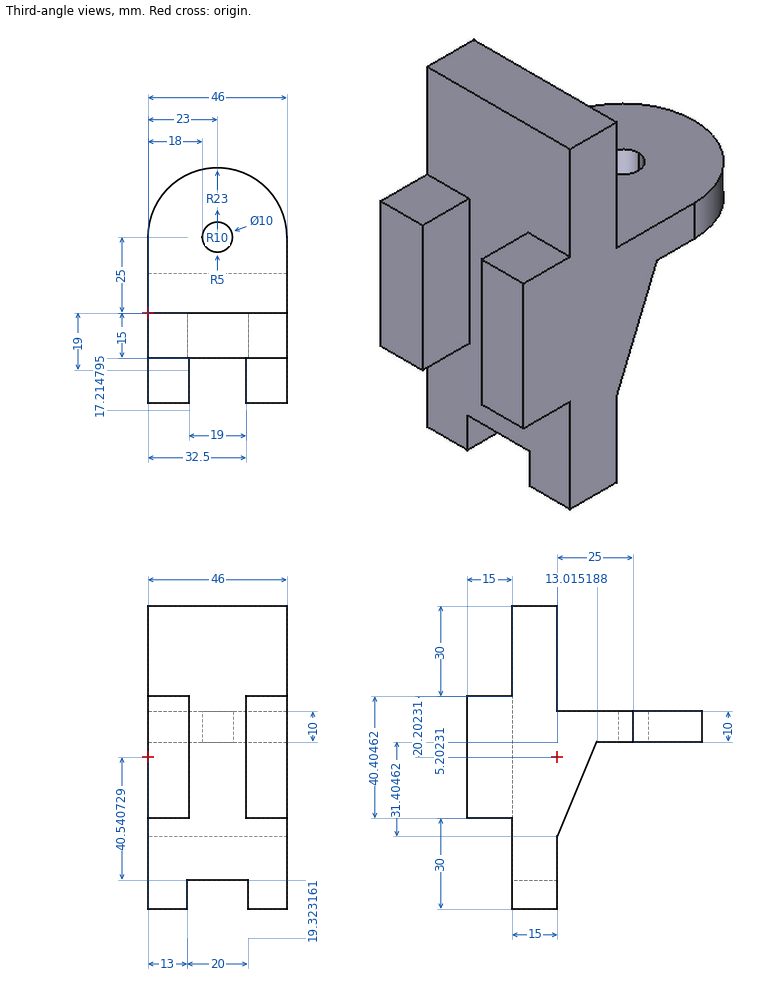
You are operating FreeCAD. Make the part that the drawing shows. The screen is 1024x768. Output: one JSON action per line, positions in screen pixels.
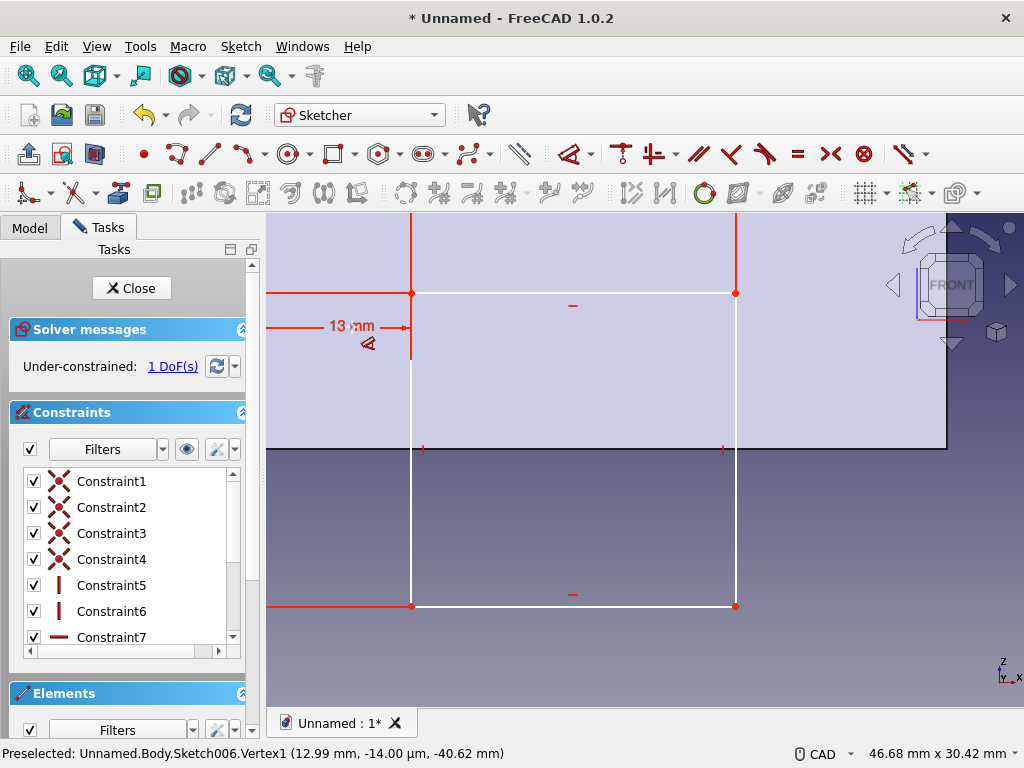
{"action": "left_click", "coordinate": [411, 293]}
{"action": "left_click", "coordinate": [445, 267]}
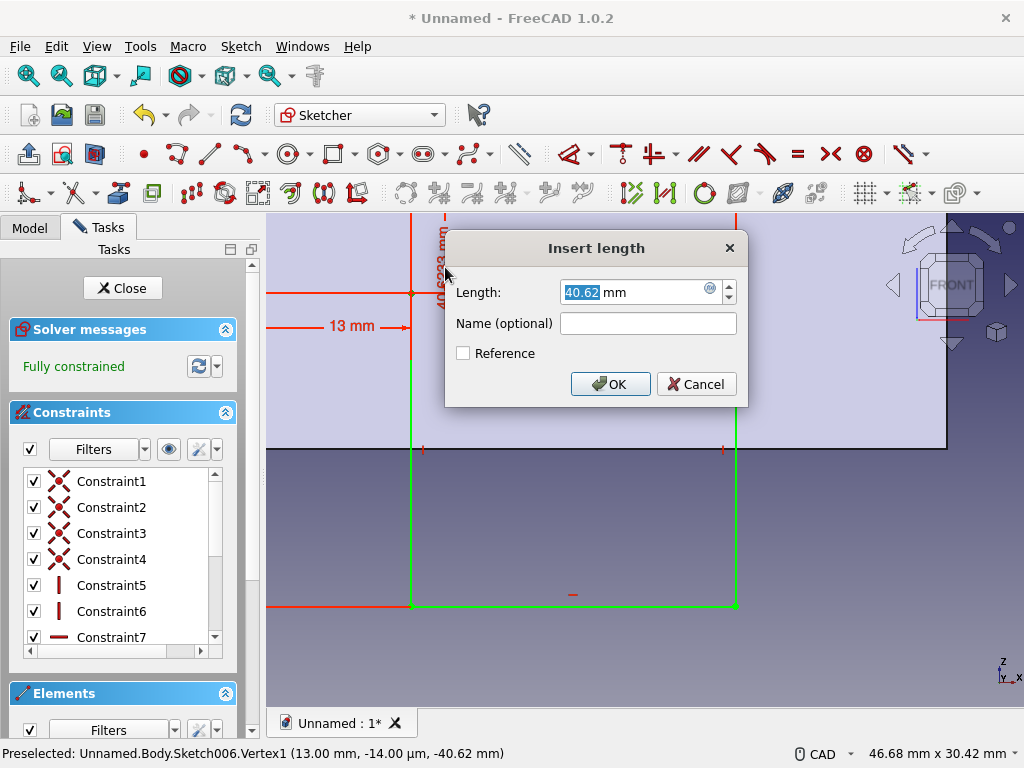
{"action": "type", "text": "40.540729"}
{"action": "key", "text": "Return"}
{"action": "key", "text": "Escape"}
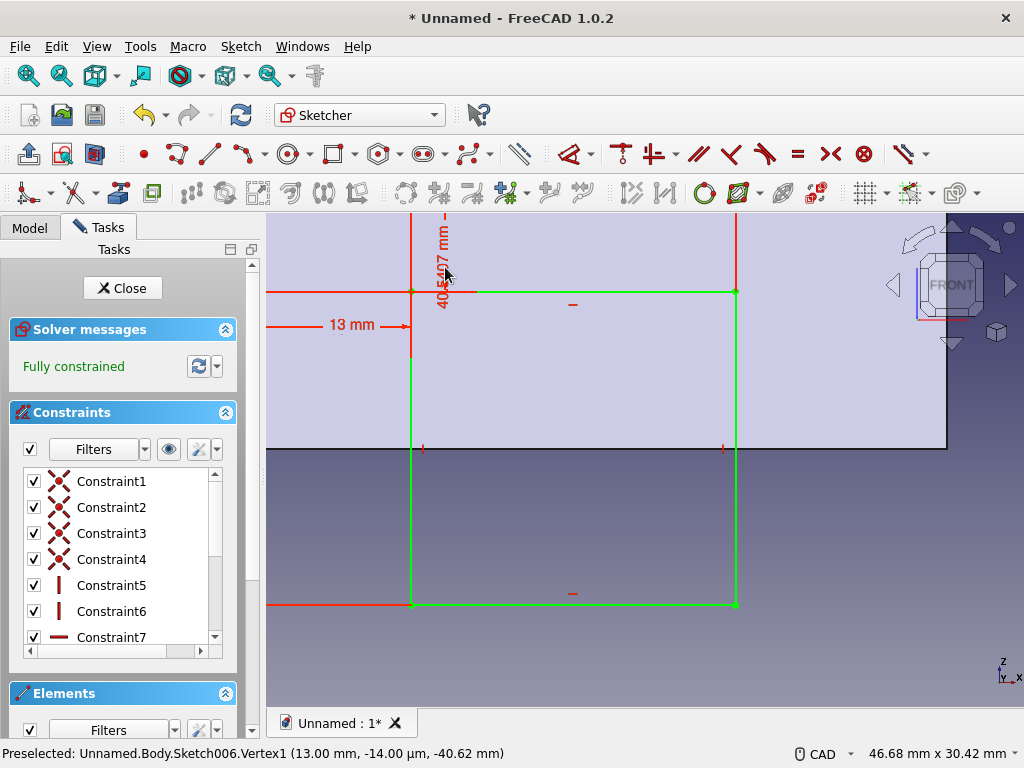
{"action": "left_click", "coordinate": [123, 288]}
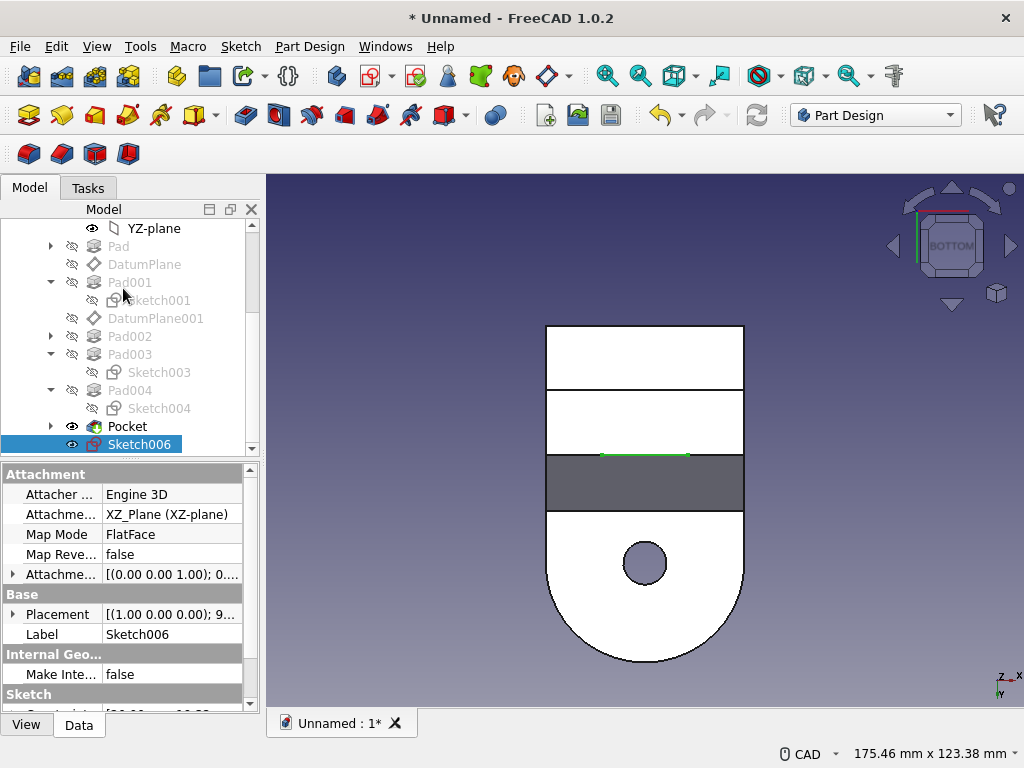
{"action": "left_click", "coordinate": [246, 116]}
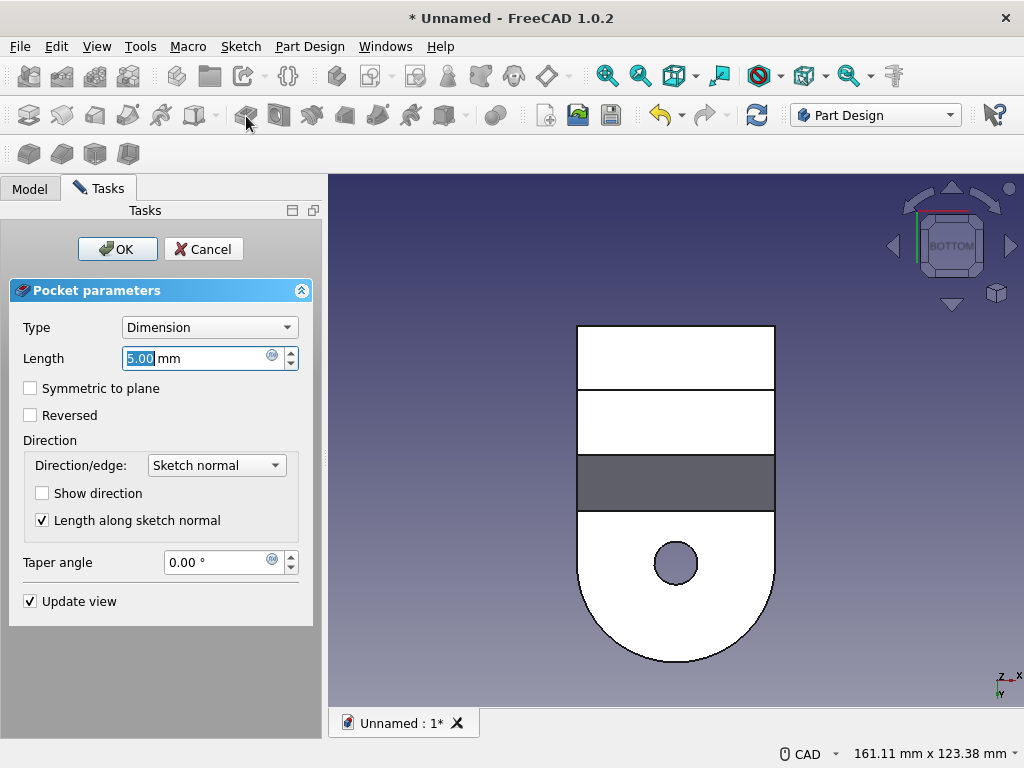
{"action": "type", "text": "19"}
{"action": "key", "text": "Tab"}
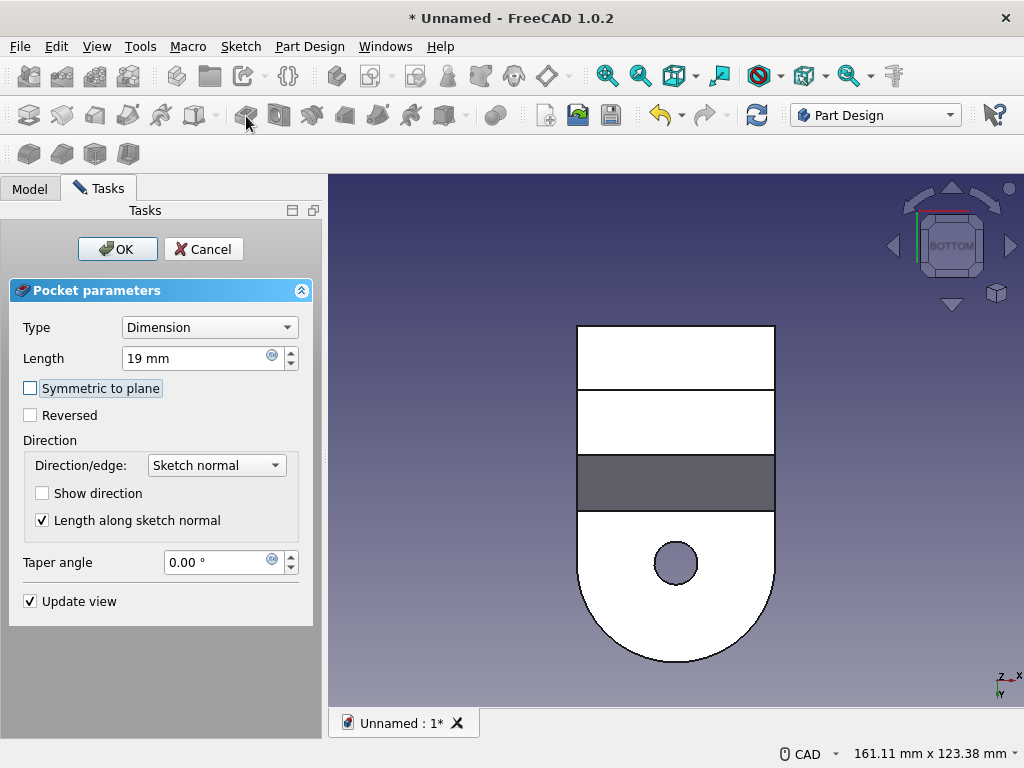
{"action": "left_click", "coordinate": [31, 415]}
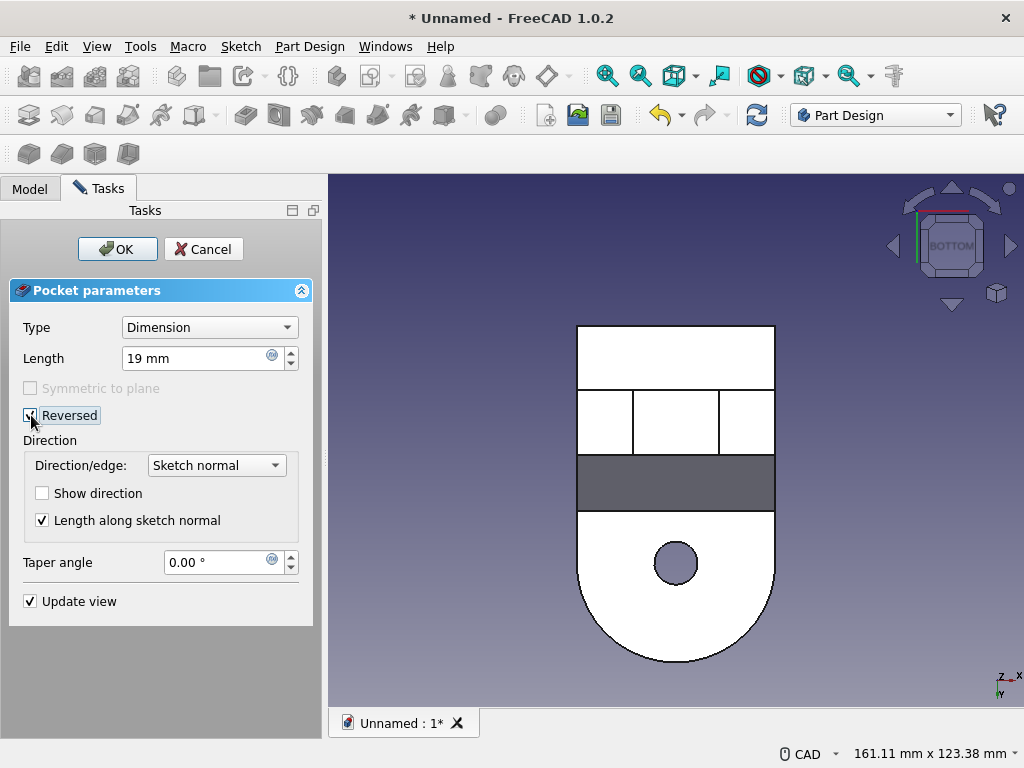
{"action": "left_click", "coordinate": [118, 249]}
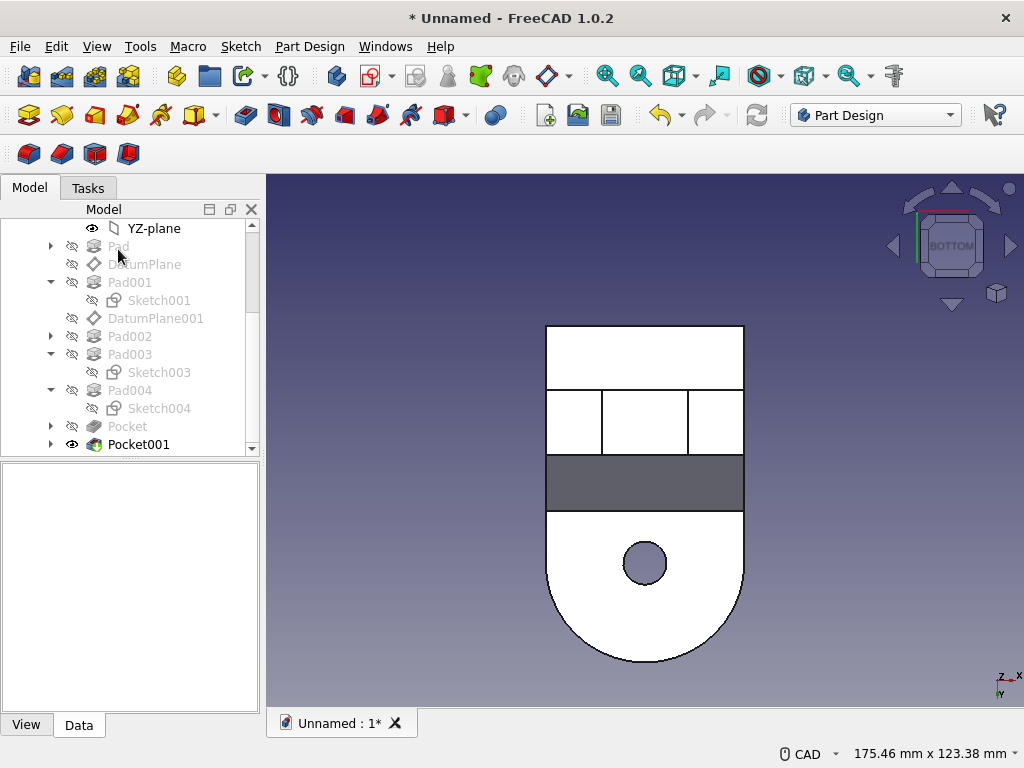
{"action": "left_click", "coordinate": [645, 357]}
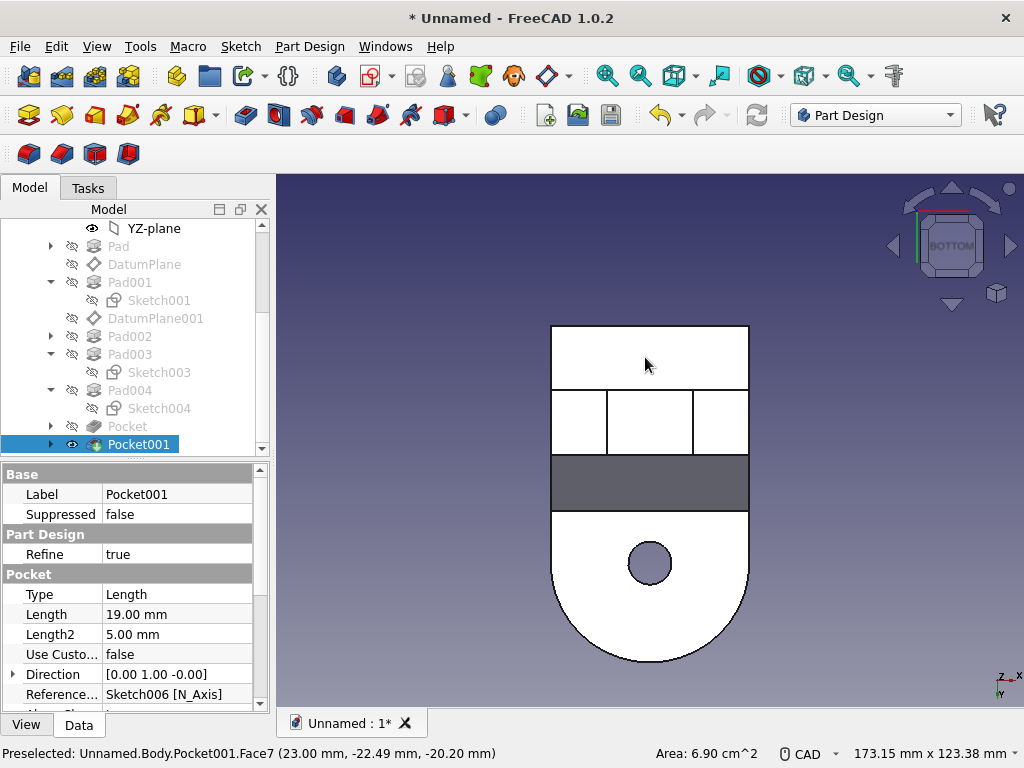
{"action": "left_click", "coordinate": [370, 76]}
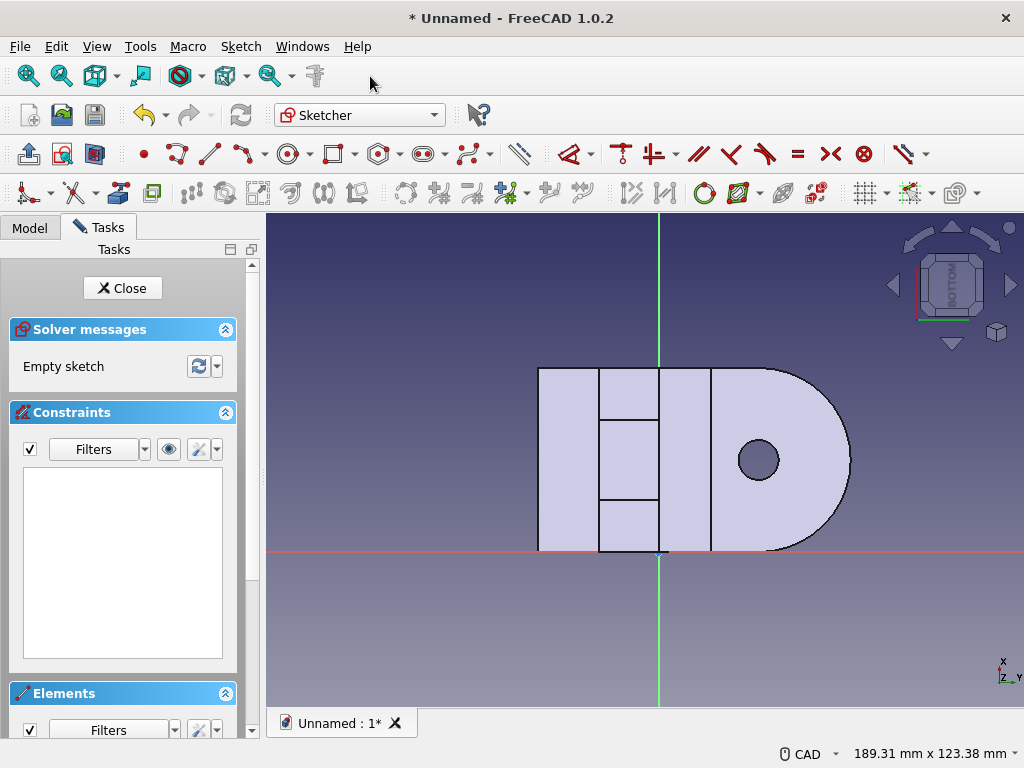
{"action": "scroll", "coordinate": [608, 509], "scroll_direction": "up", "scroll_amount": 4}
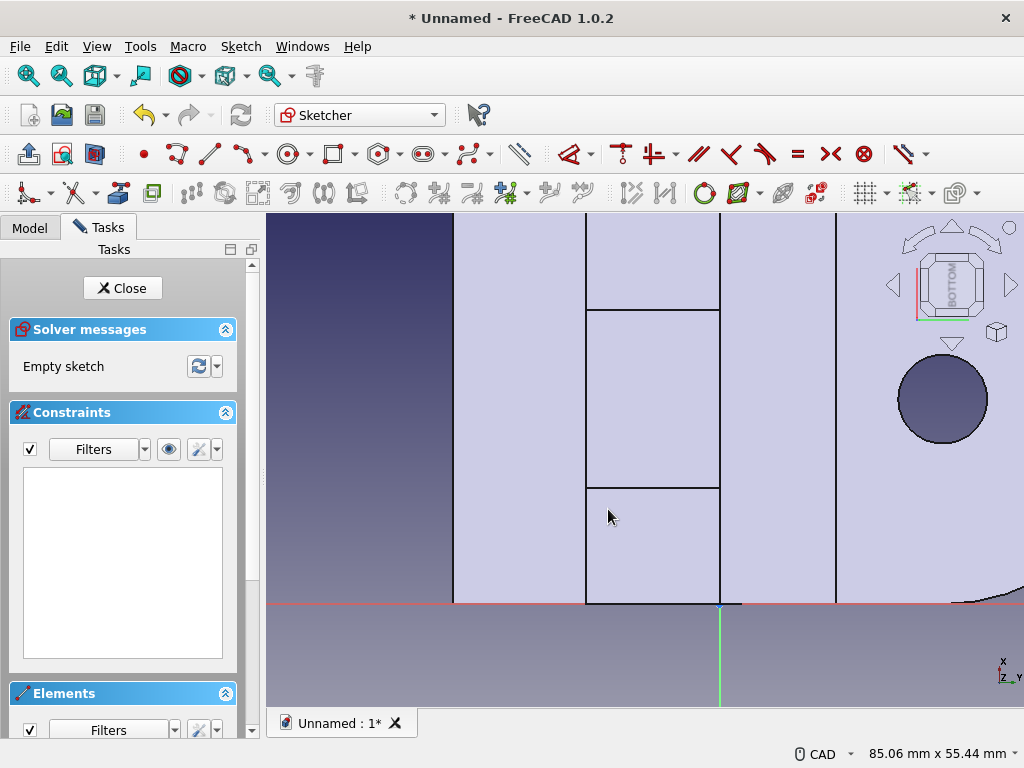
{"action": "key", "text": "g r"}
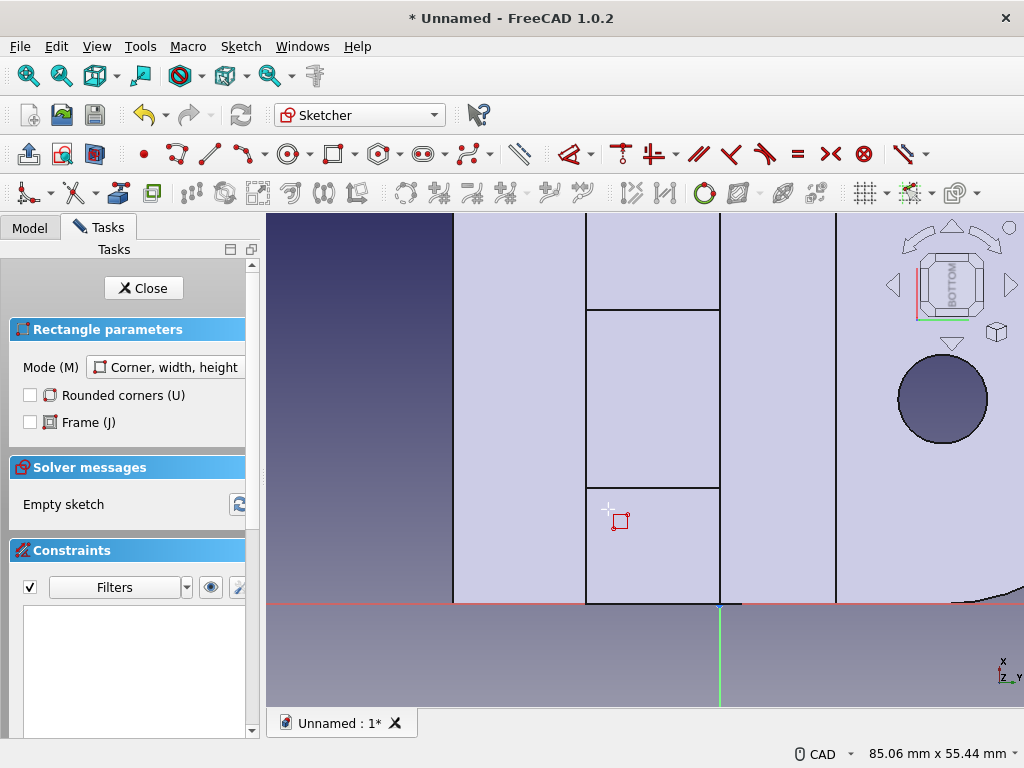
{"action": "left_click", "coordinate": [433, 315]}
{"action": "mouse_move", "coordinate": [586, 484]}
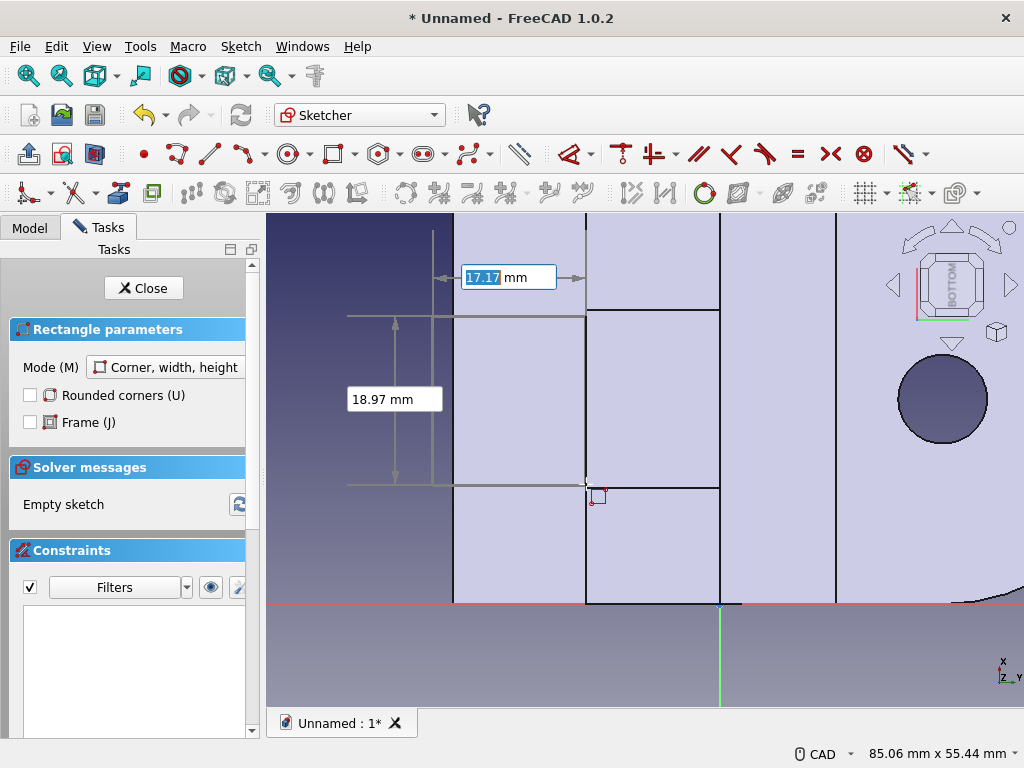
{"action": "type", "text": "17.214795"}
{"action": "key", "text": "Tab"}
{"action": "type", "text": "19"}
{"action": "key", "text": "Return"}
{"action": "key", "text": "Escape"}